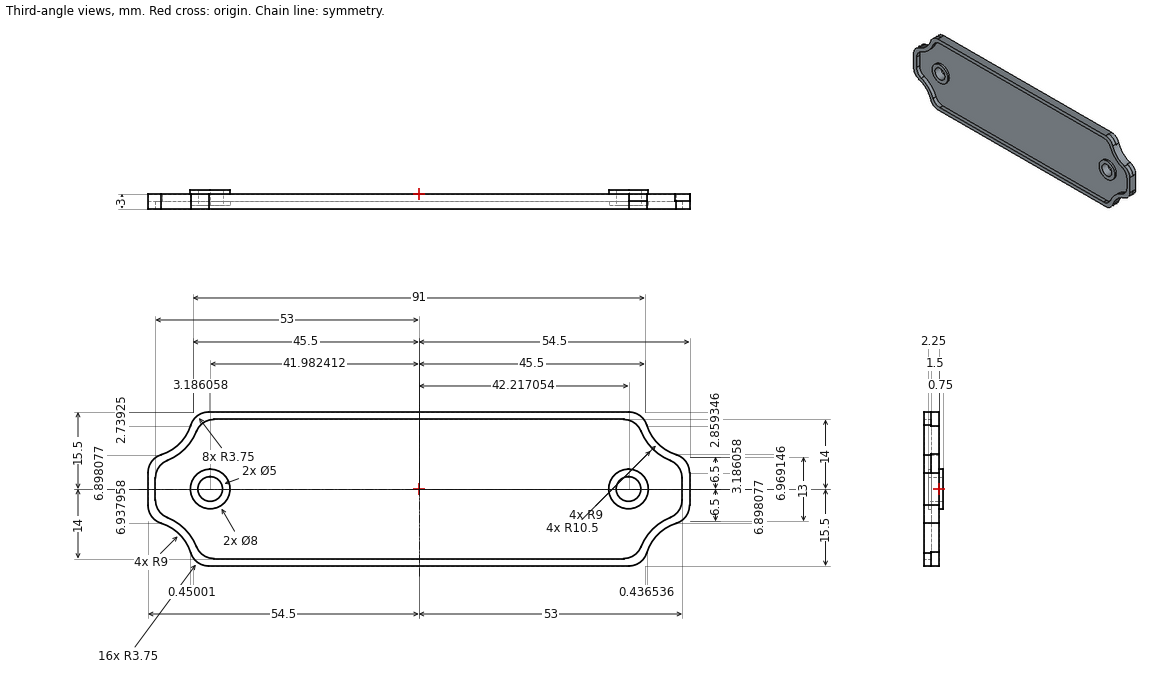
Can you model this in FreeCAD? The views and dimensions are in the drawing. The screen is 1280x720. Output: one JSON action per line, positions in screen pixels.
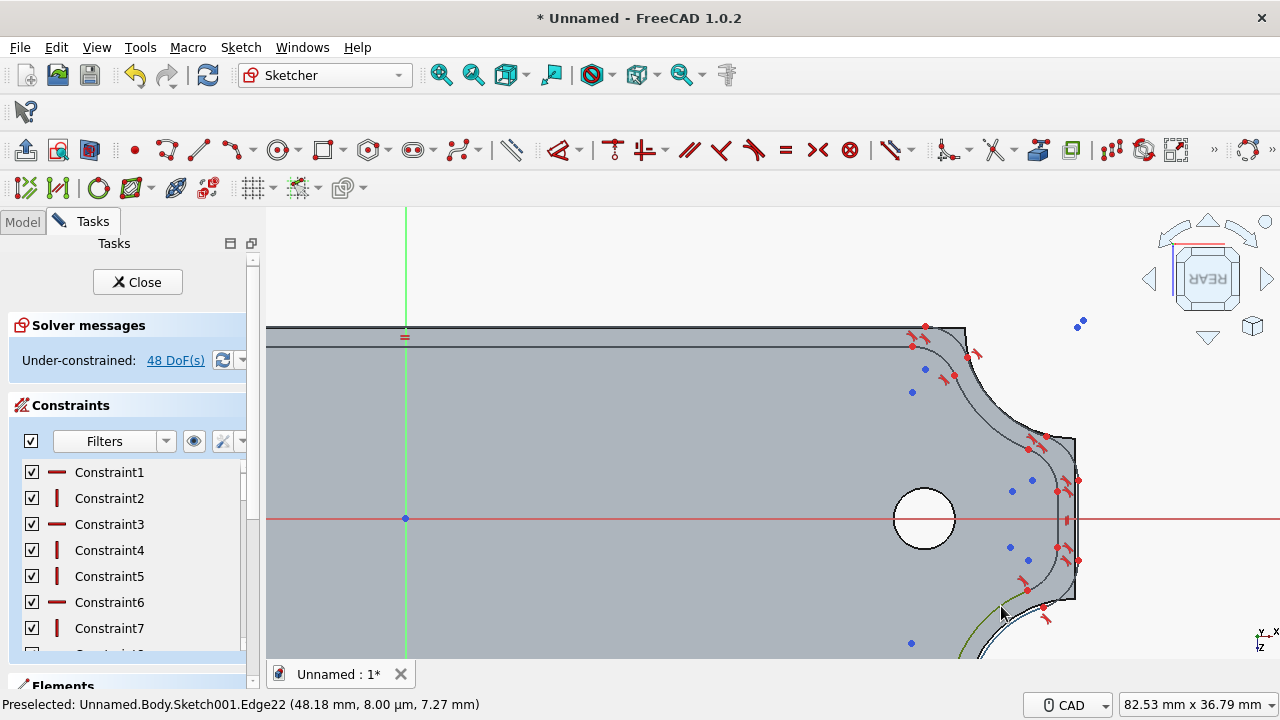
{"action": "left_click", "coordinate": [614, 150]}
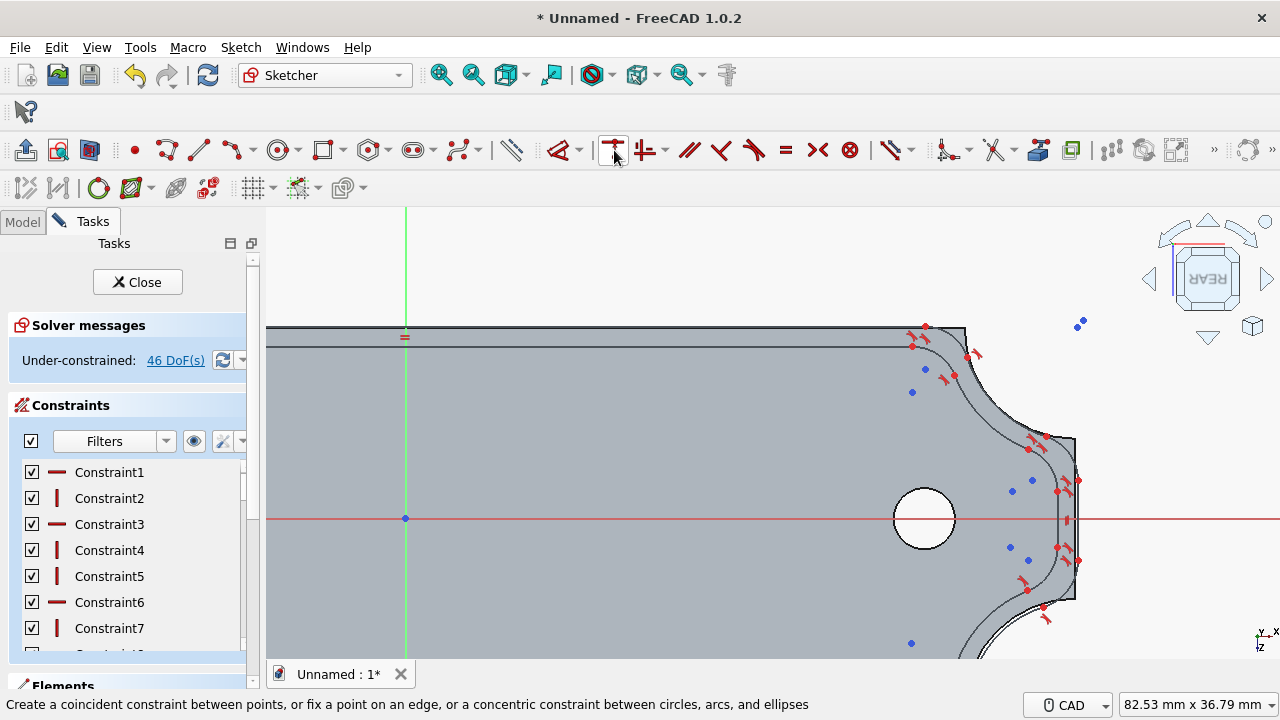
{"action": "scroll", "coordinate": [948, 363], "scroll_direction": "down", "scroll_amount": 4}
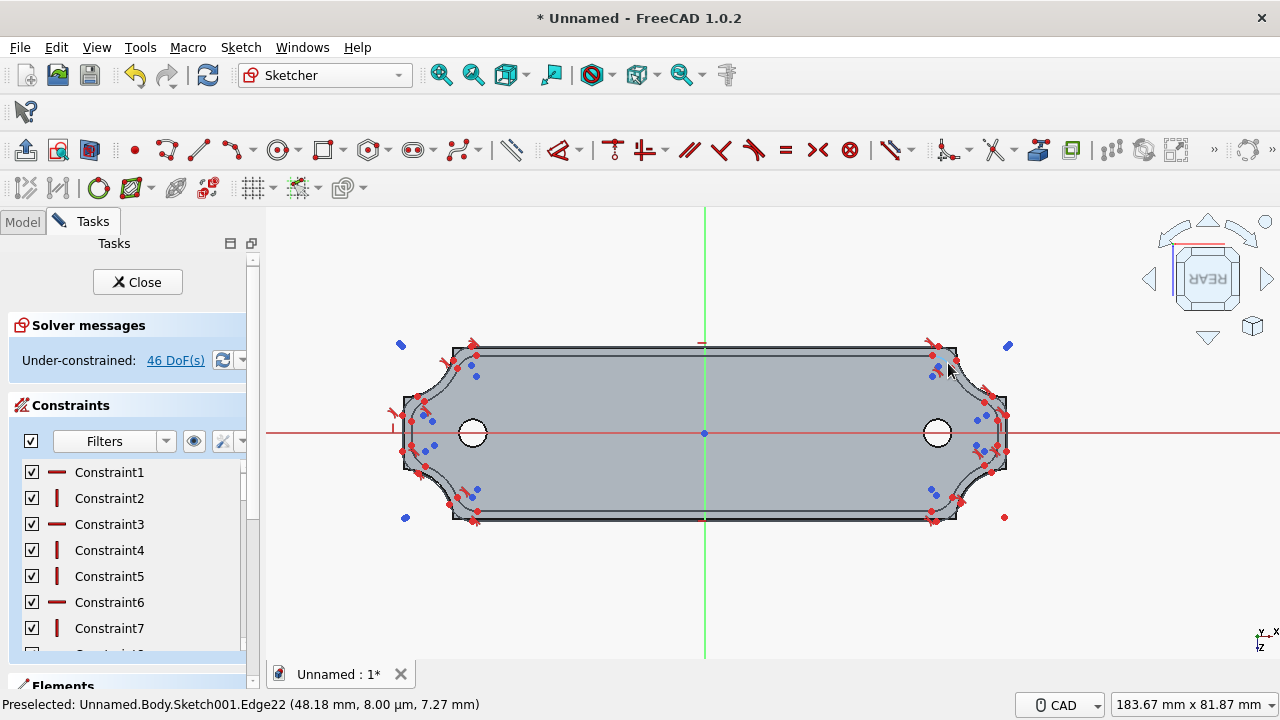
{"action": "scroll", "coordinate": [444, 492], "scroll_direction": "up", "scroll_amount": 2}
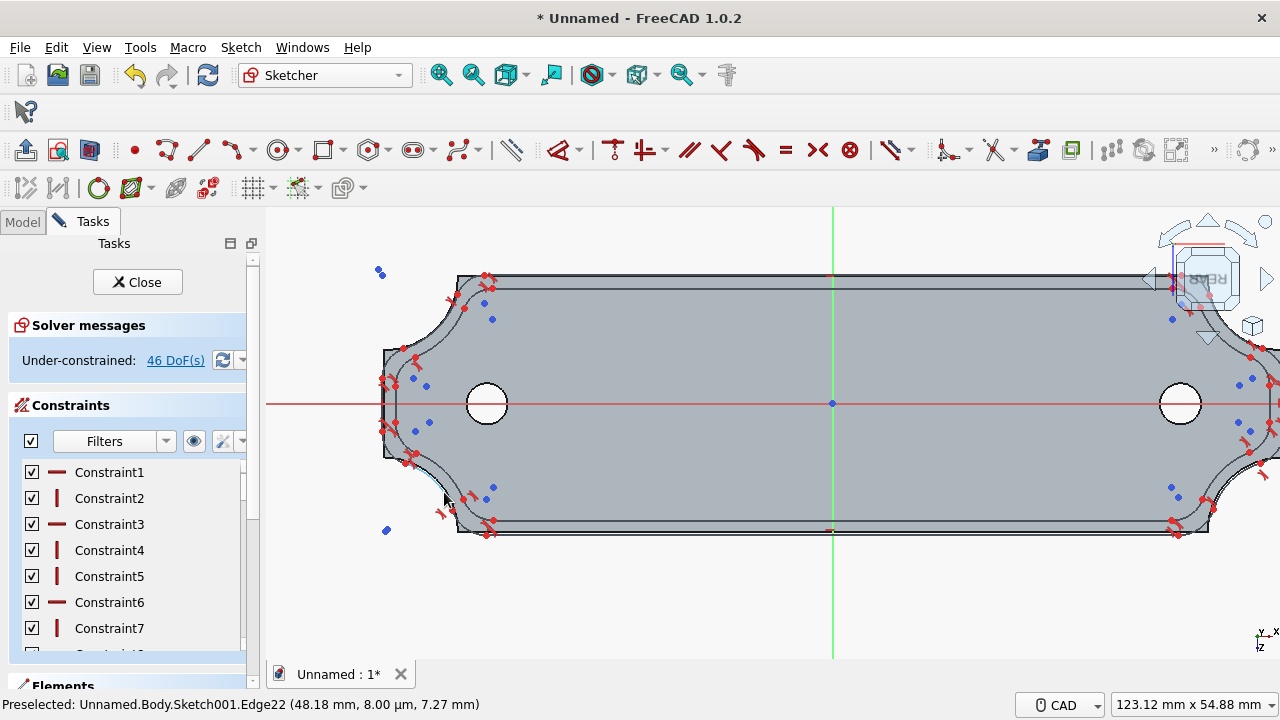
{"action": "left_click", "coordinate": [444, 492]}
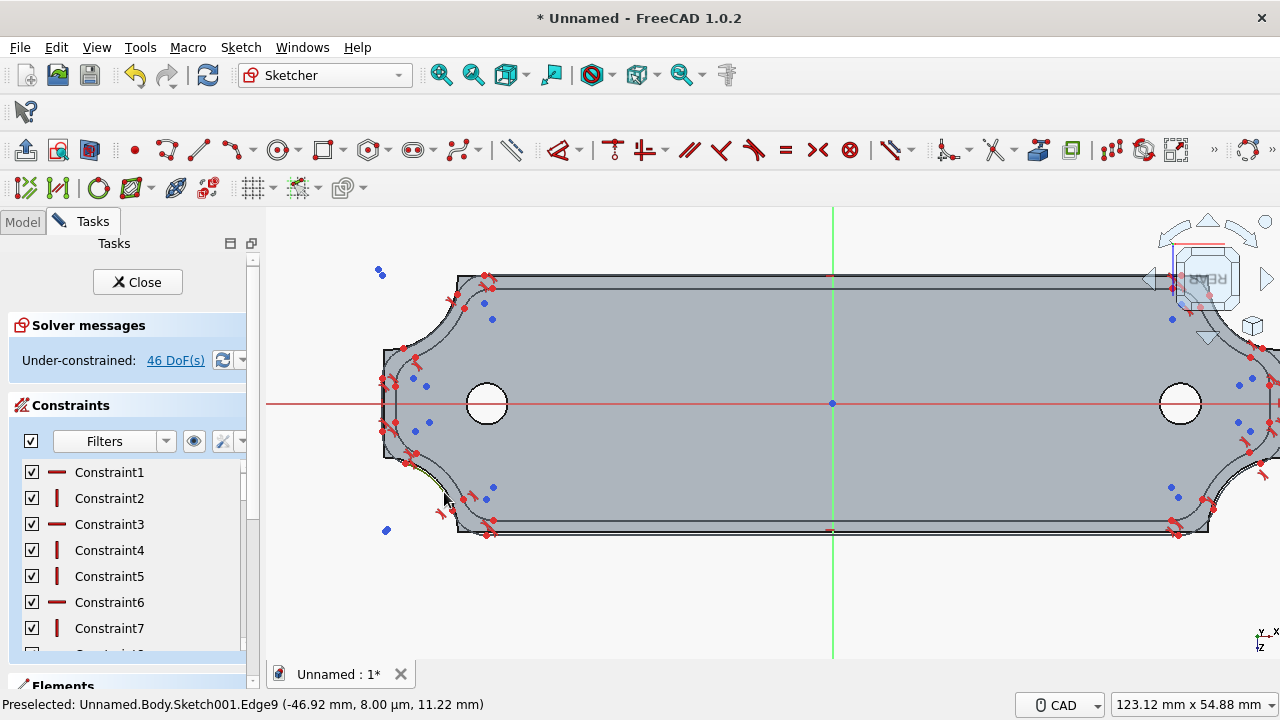
{"action": "left_click", "coordinate": [454, 482]}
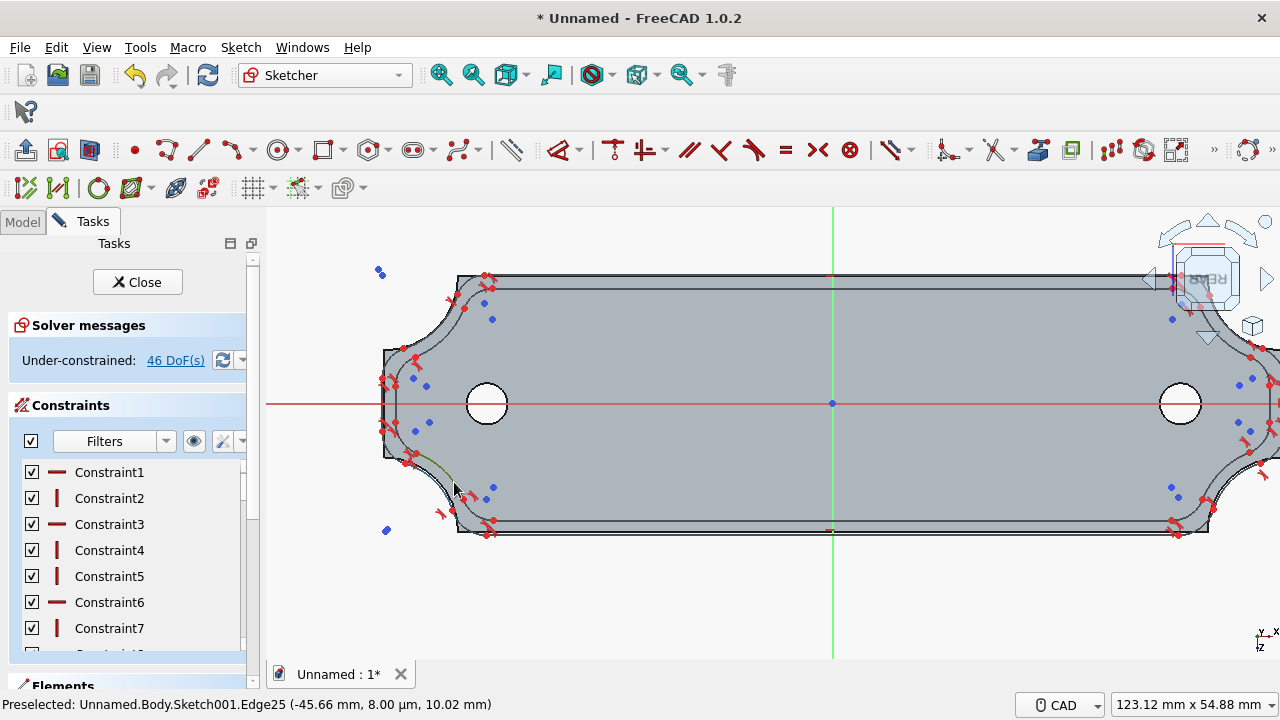
{"action": "left_click", "coordinate": [614, 150]}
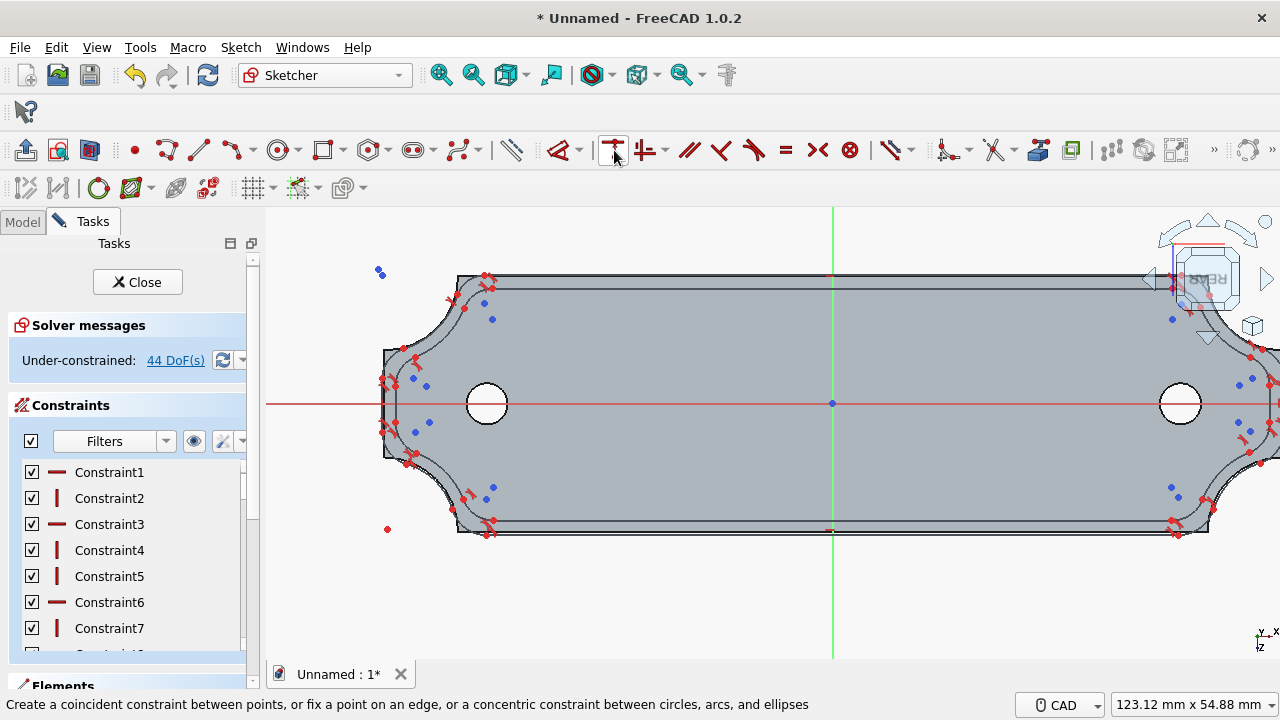
{"action": "left_click", "coordinate": [425, 339]}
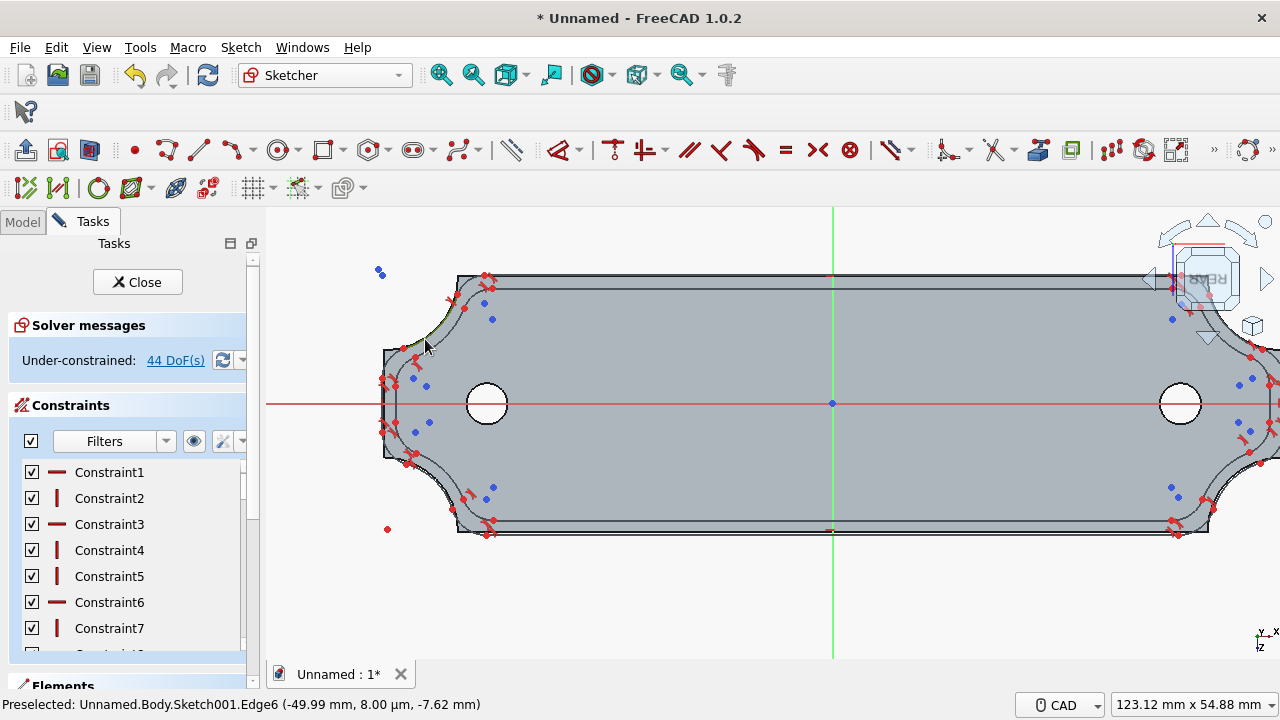
{"action": "left_click", "coordinate": [434, 347]}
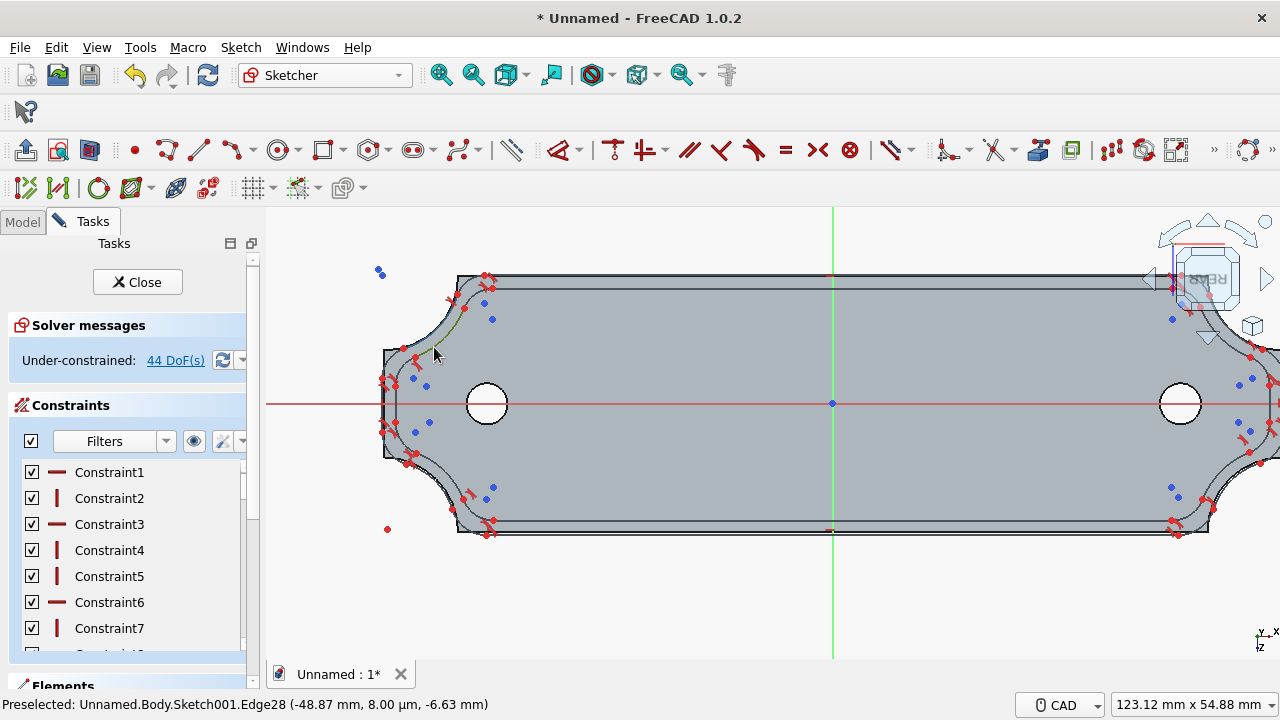
{"action": "left_click", "coordinate": [614, 150]}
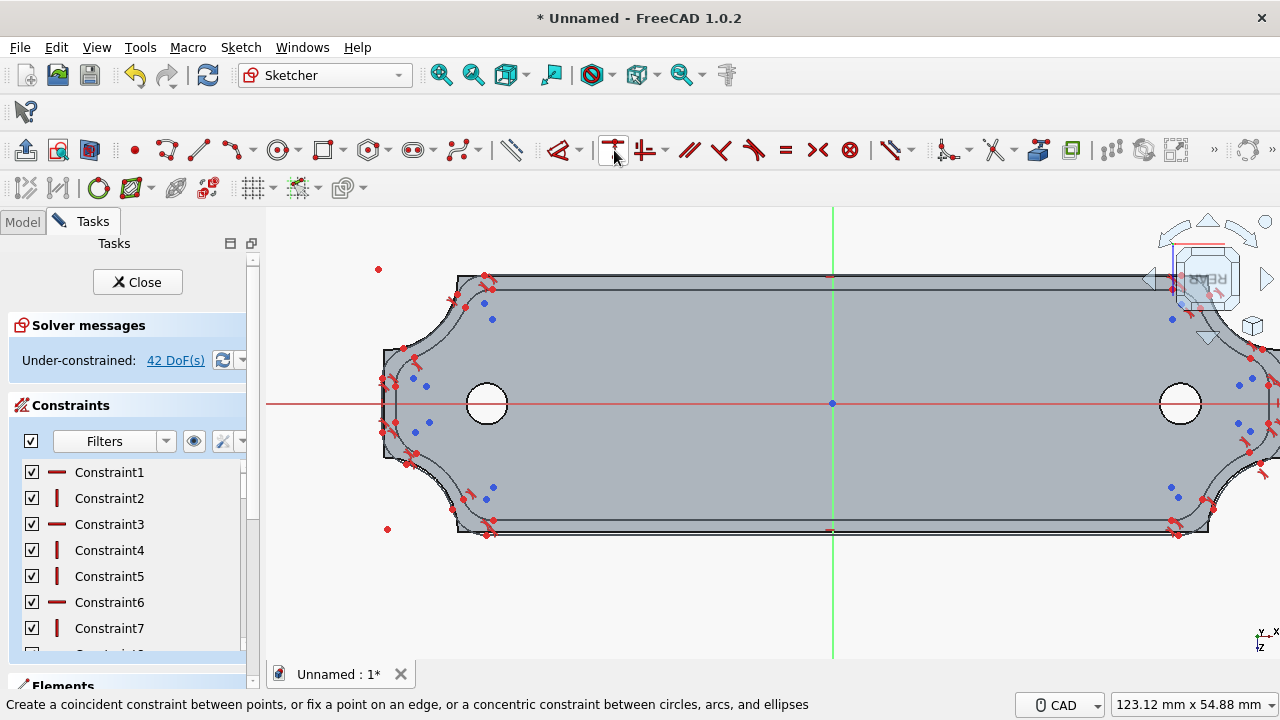
{"action": "scroll", "coordinate": [444, 492], "scroll_direction": "down", "scroll_amount": 2}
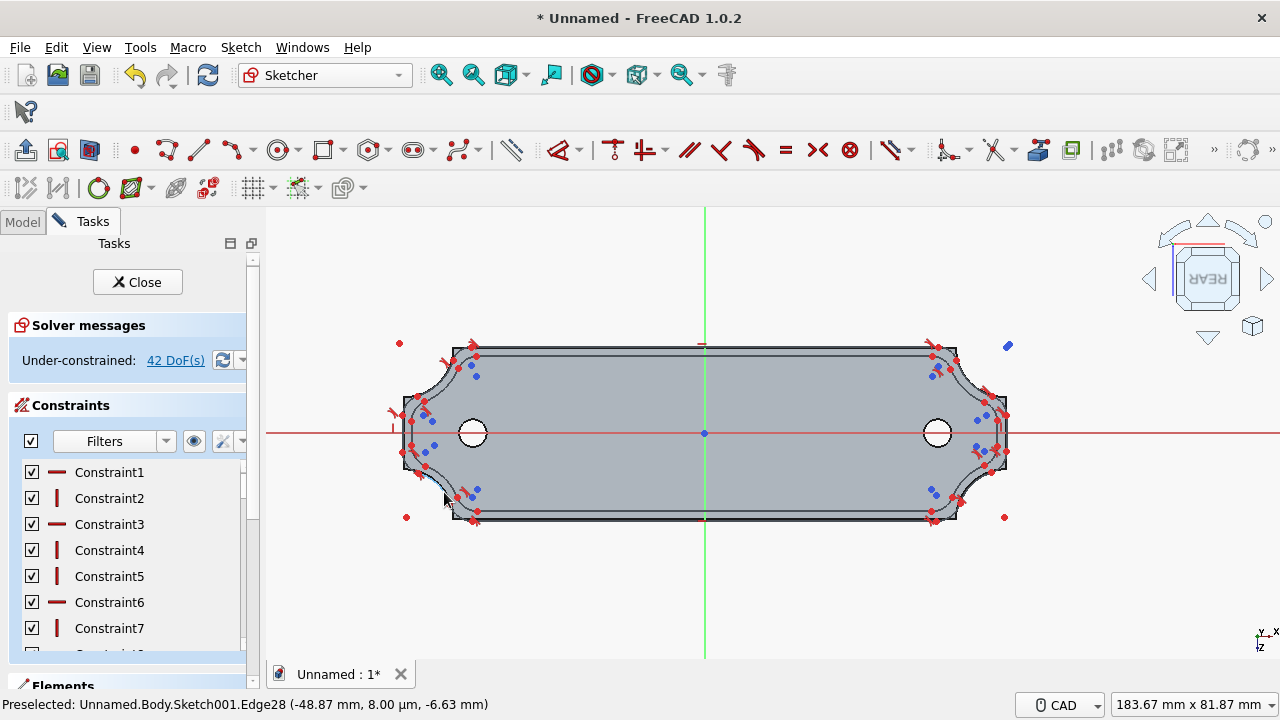
{"action": "scroll", "coordinate": [964, 375], "scroll_direction": "up", "scroll_amount": 3}